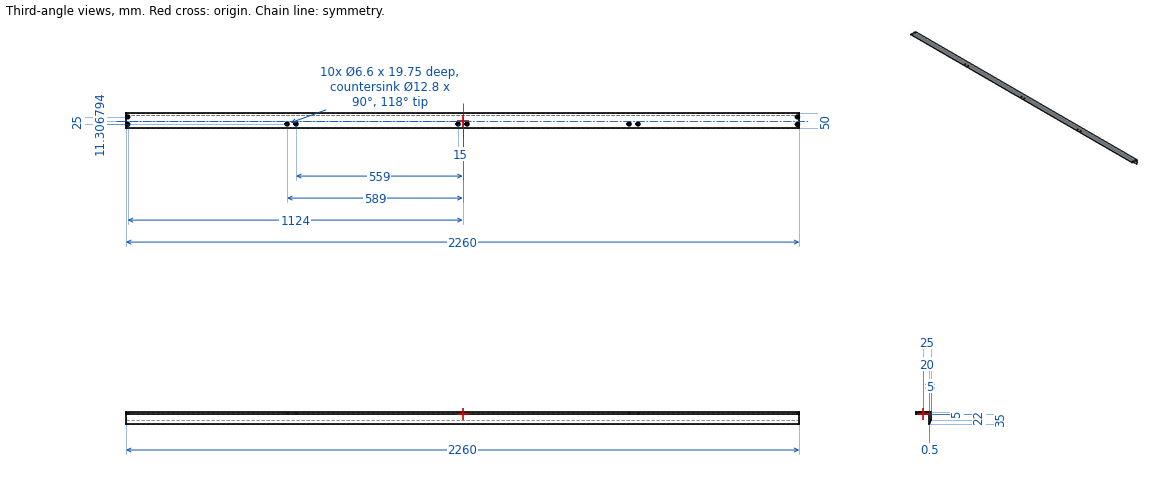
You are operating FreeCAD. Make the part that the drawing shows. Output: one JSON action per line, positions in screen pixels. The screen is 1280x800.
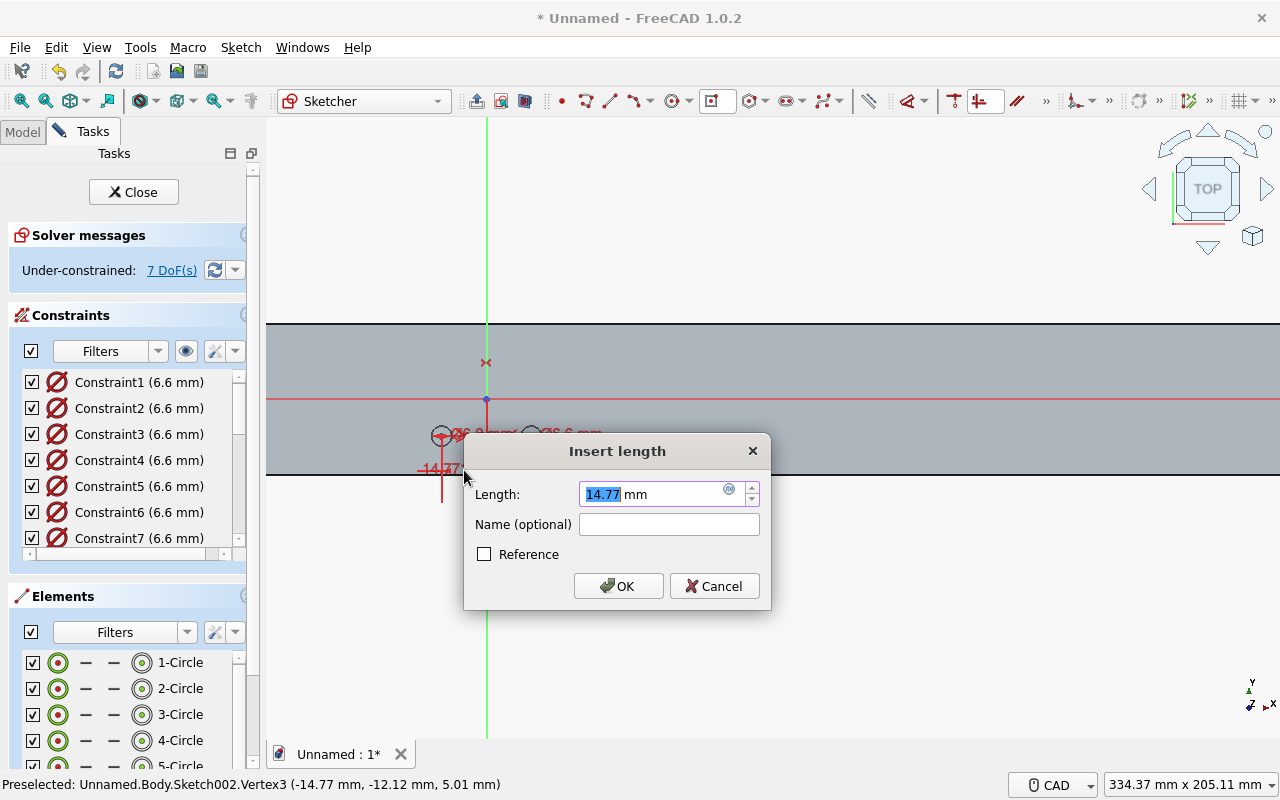
{"action": "type", "text": "15"}
{"action": "key", "text": "Return"}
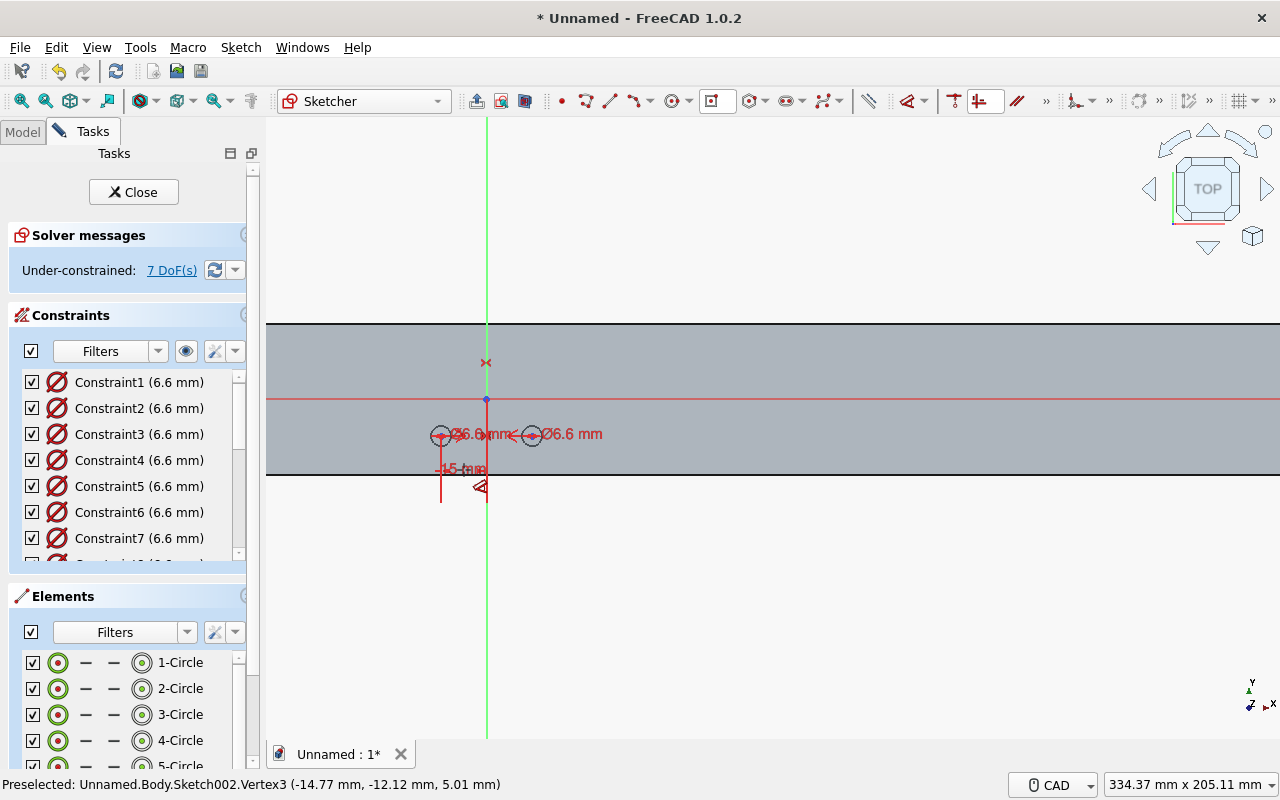
{"action": "scroll", "coordinate": [726, 431], "scroll_direction": "down", "scroll_amount": 12}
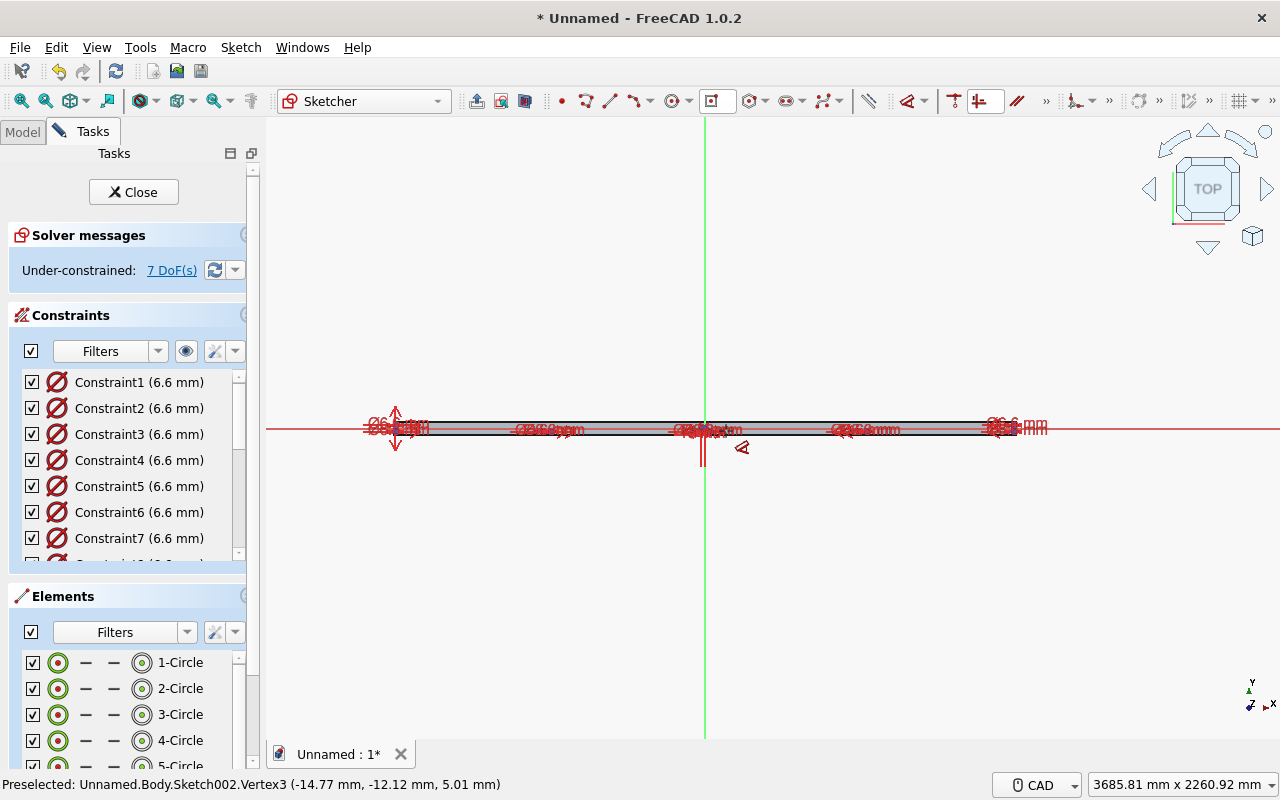
{"action": "scroll", "coordinate": [543, 432], "scroll_direction": "up", "scroll_amount": 2}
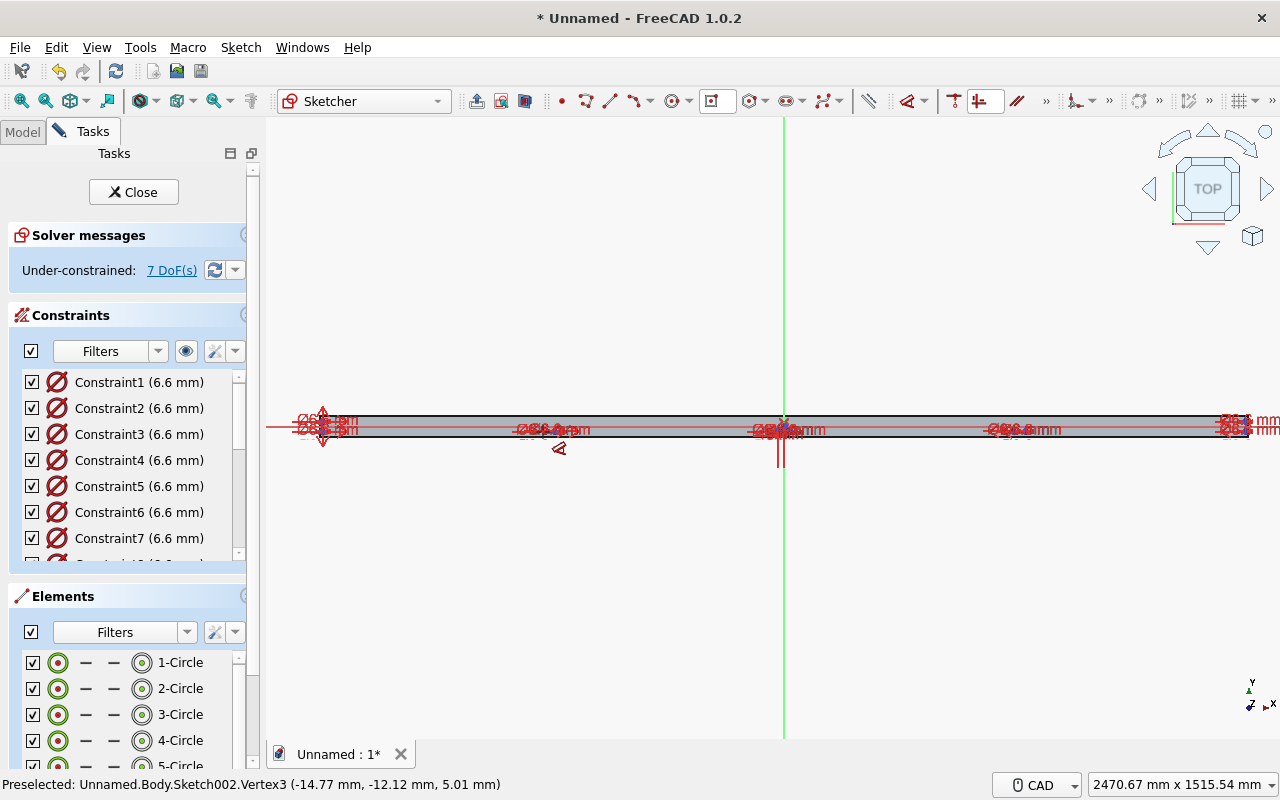
{"action": "left_click", "coordinate": [542, 432]}
{"action": "left_click", "coordinate": [663, 466]}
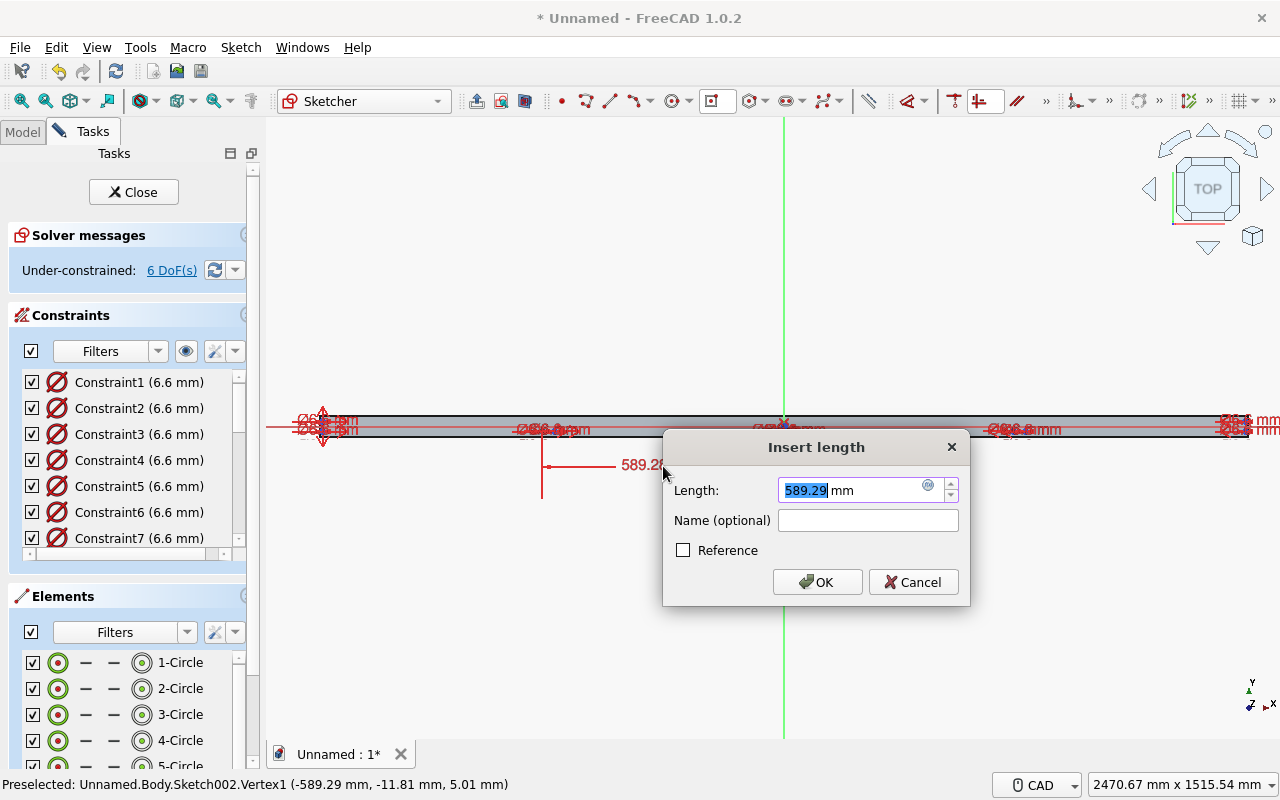
{"action": "type", "text": "589"}
{"action": "key", "text": "Return"}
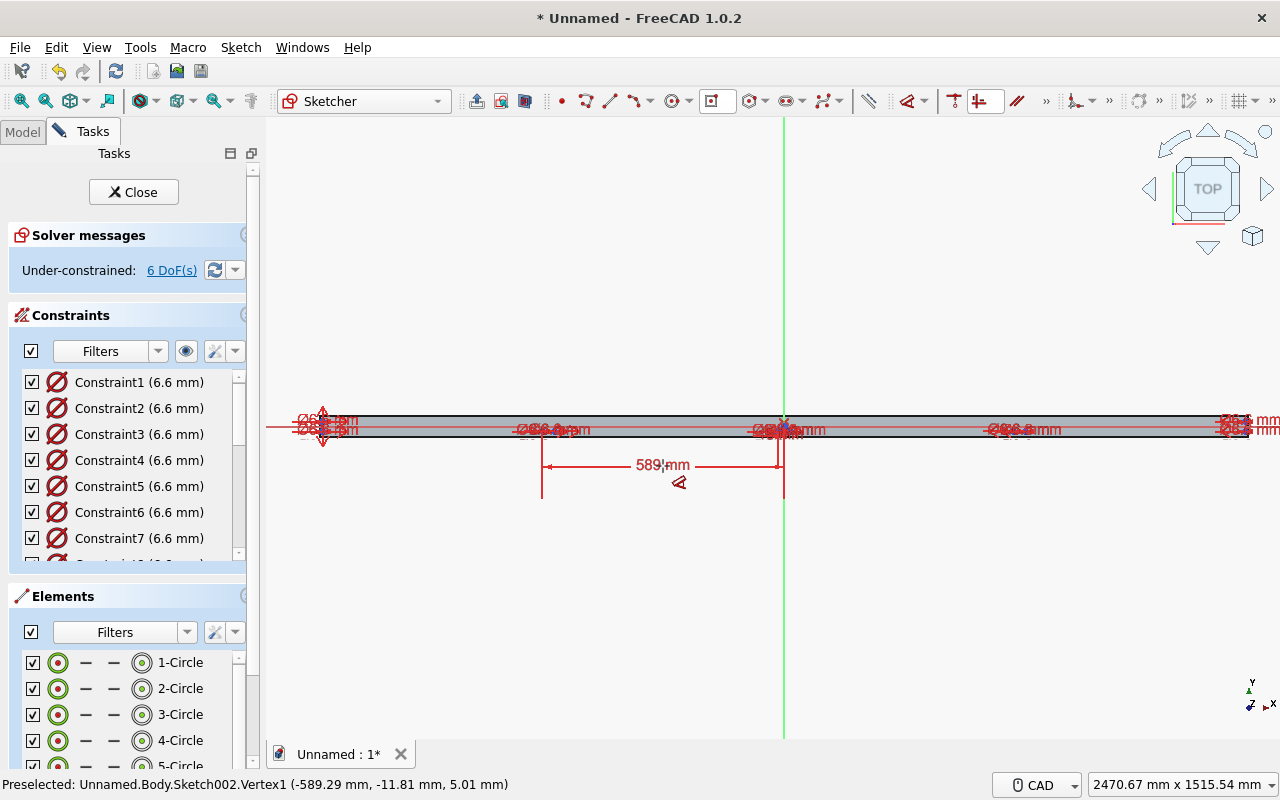
{"action": "left_click", "coordinate": [555, 431]}
{"action": "left_click", "coordinate": [589, 465]}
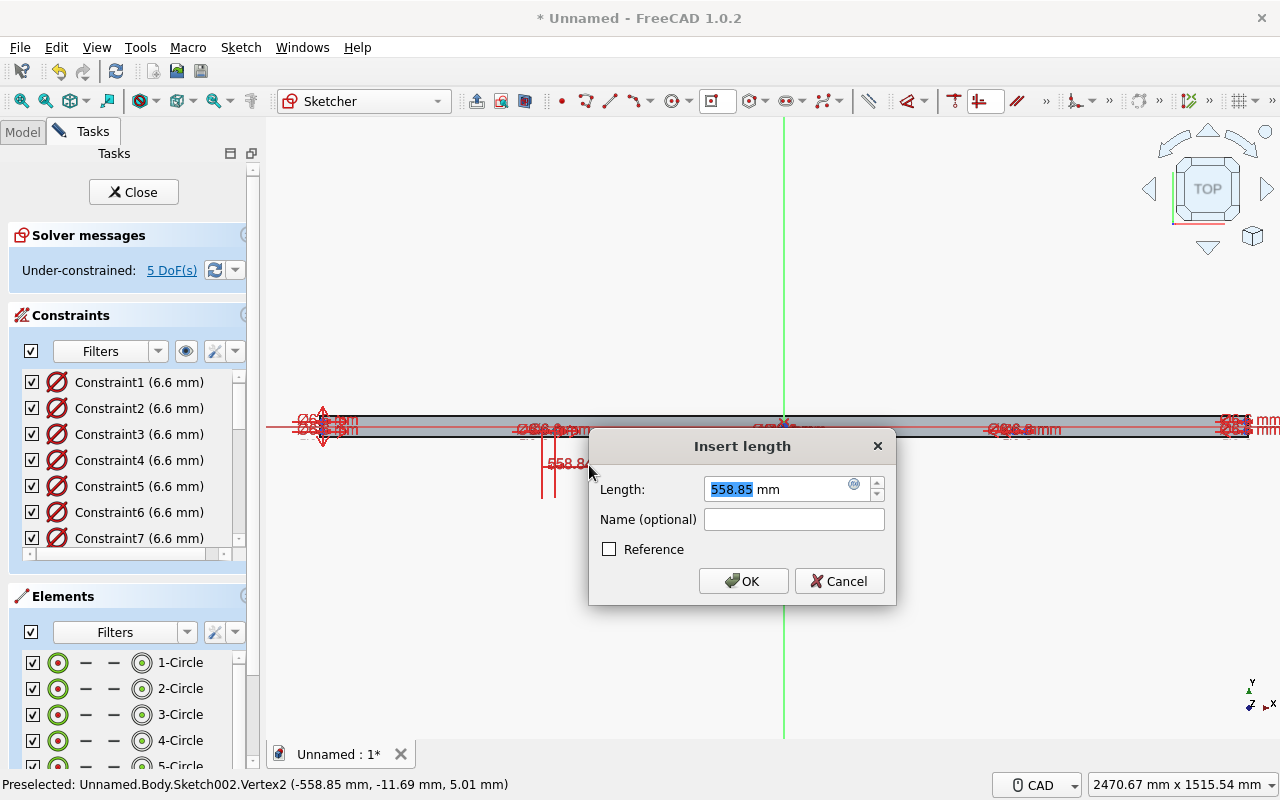
{"action": "type", "text": "559"}
{"action": "key", "text": "Return"}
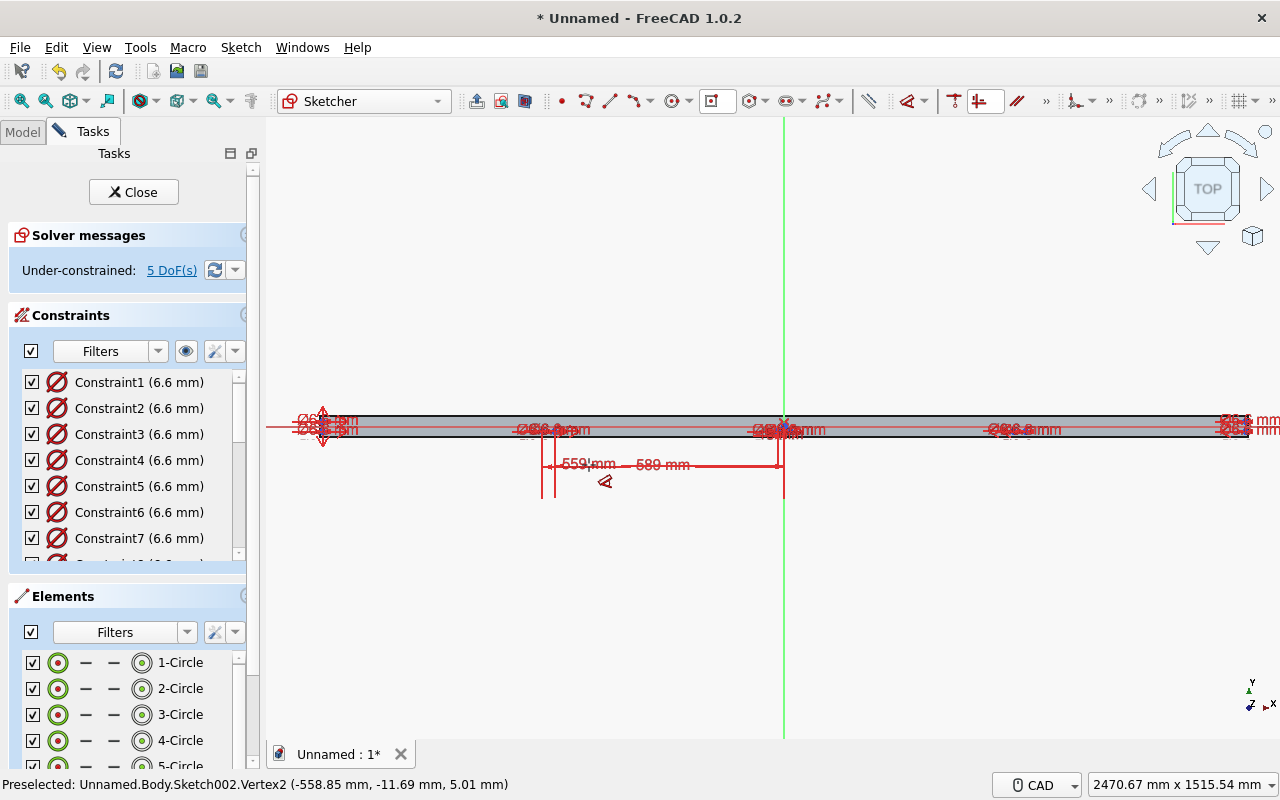
{"action": "scroll", "coordinate": [323, 432], "scroll_direction": "up", "scroll_amount": 7}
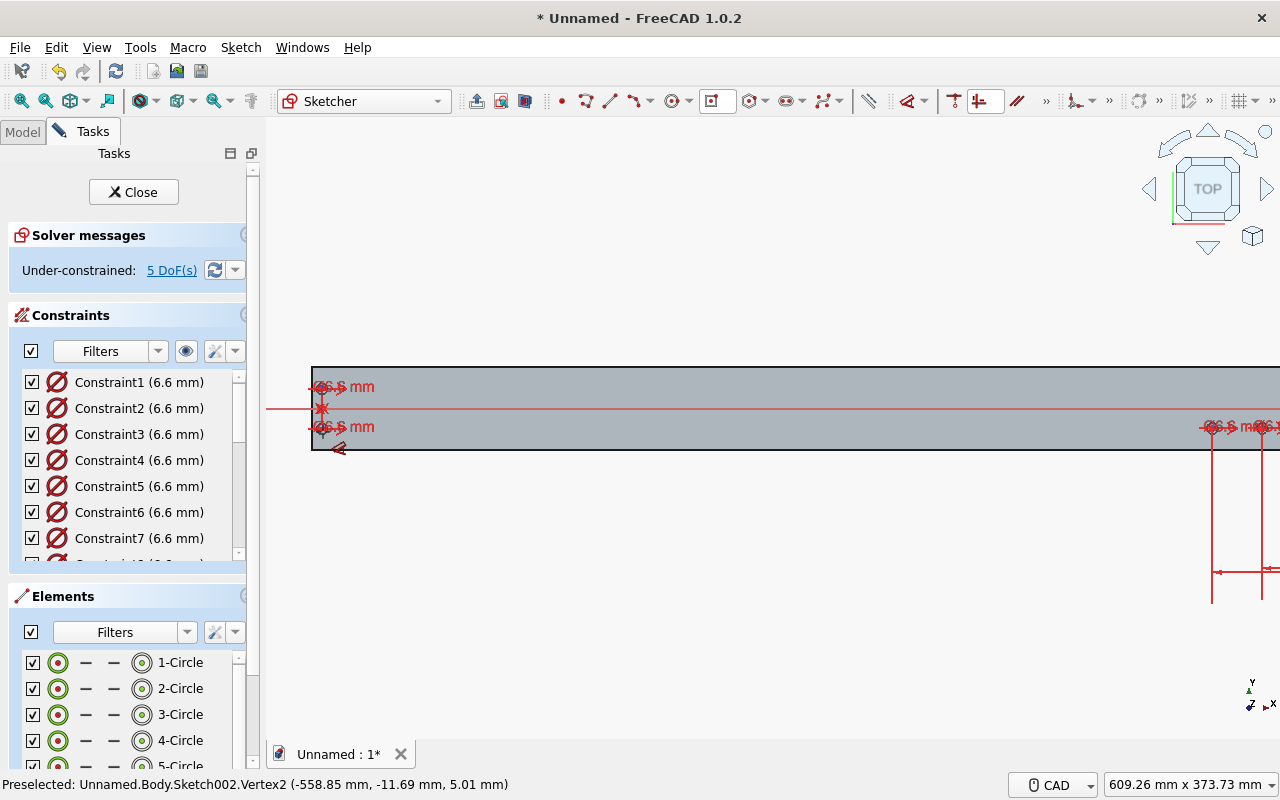
{"action": "left_click", "coordinate": [322, 429]}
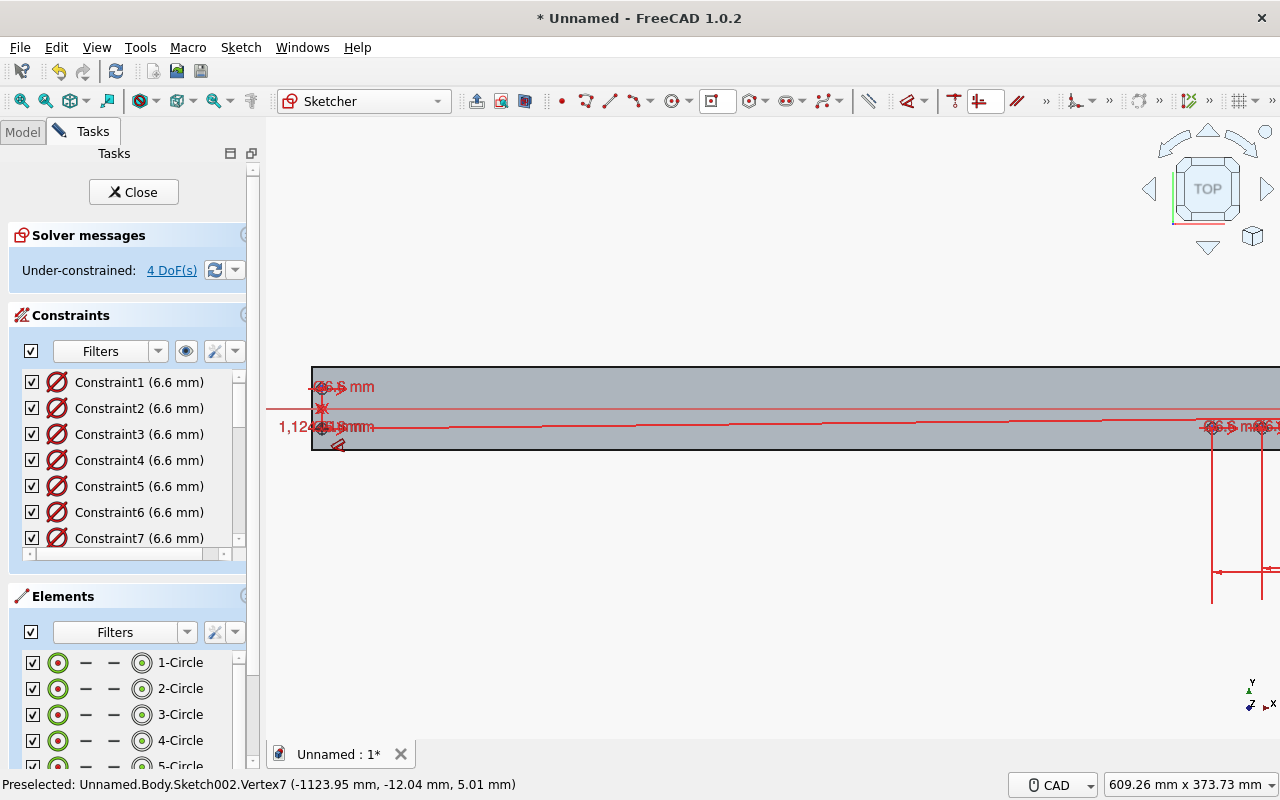
{"action": "left_click", "coordinate": [322, 389]}
{"action": "left_click", "coordinate": [356, 395]}